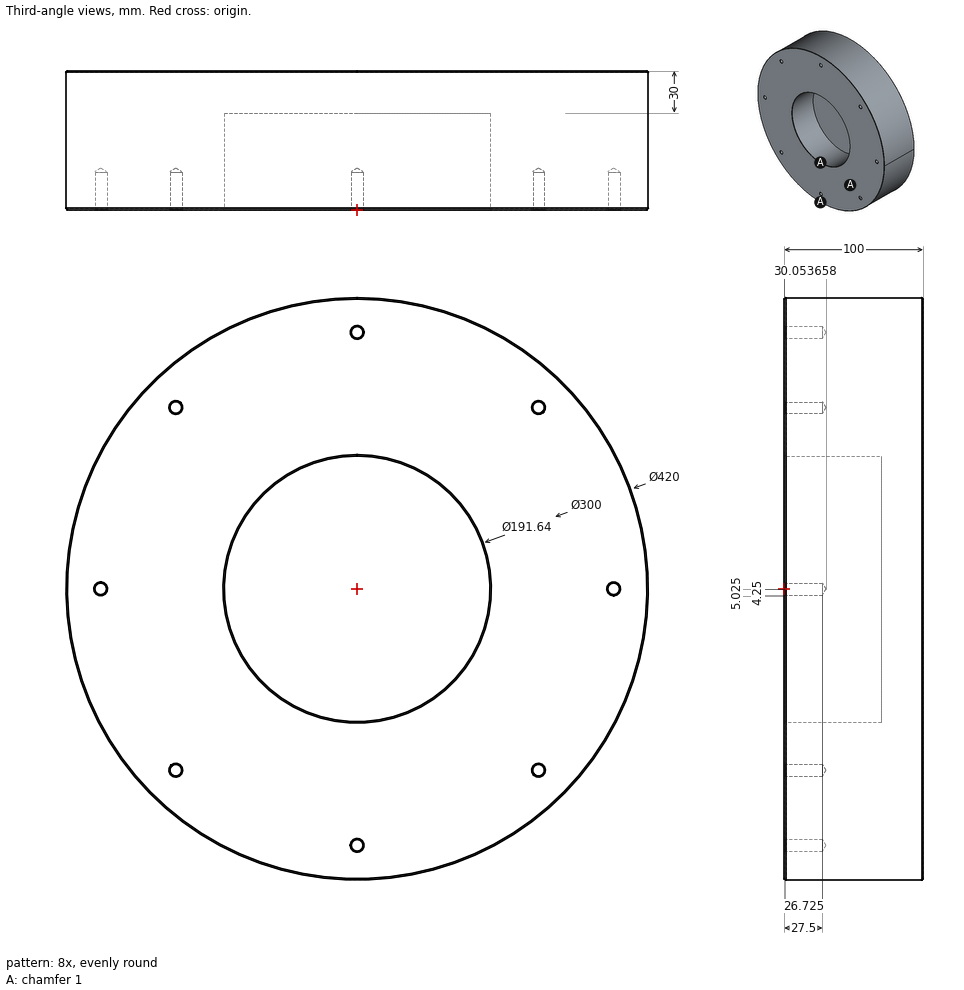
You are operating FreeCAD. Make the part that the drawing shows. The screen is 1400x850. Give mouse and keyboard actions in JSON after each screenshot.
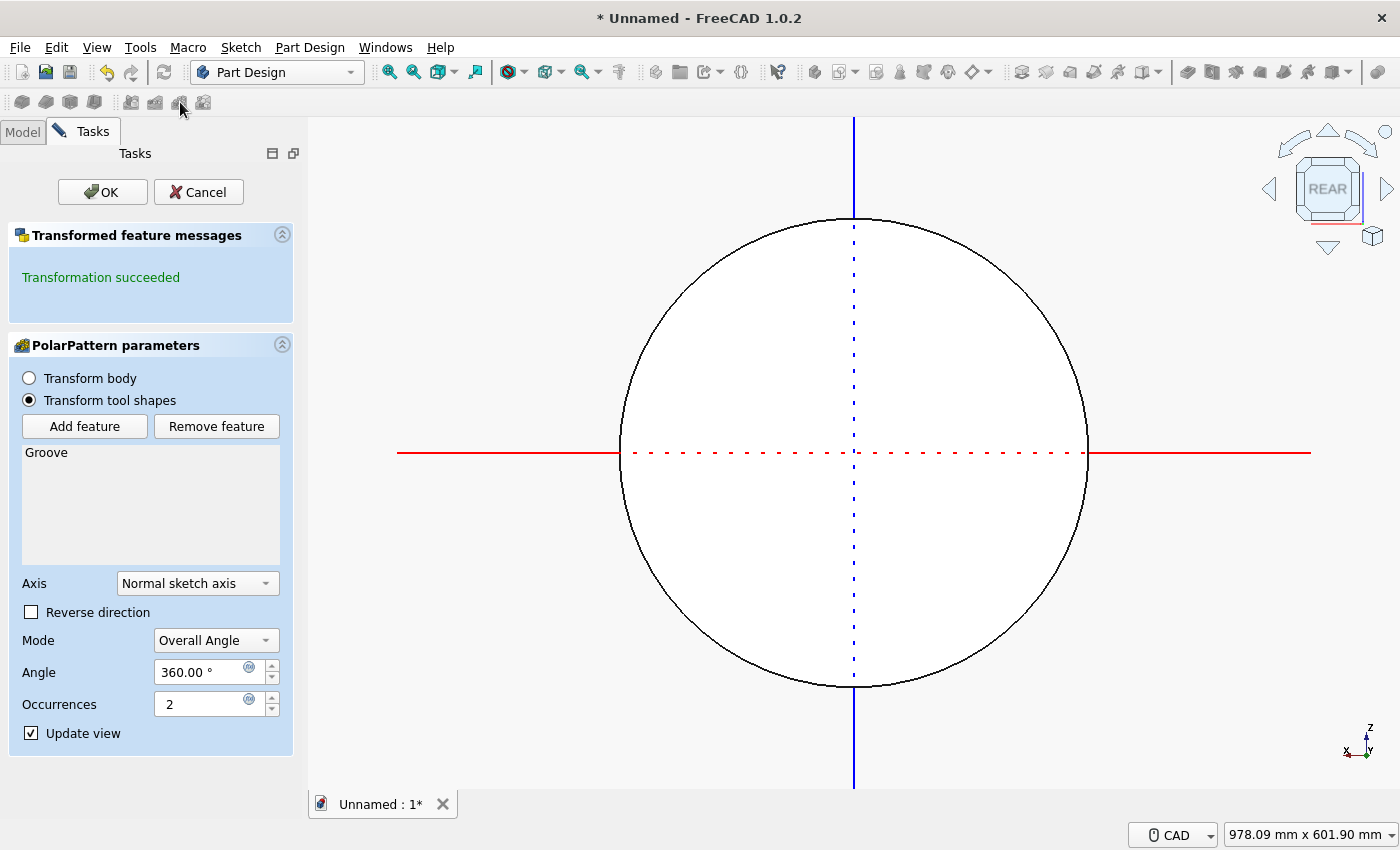
{"action": "left_click", "coordinate": [198, 584]}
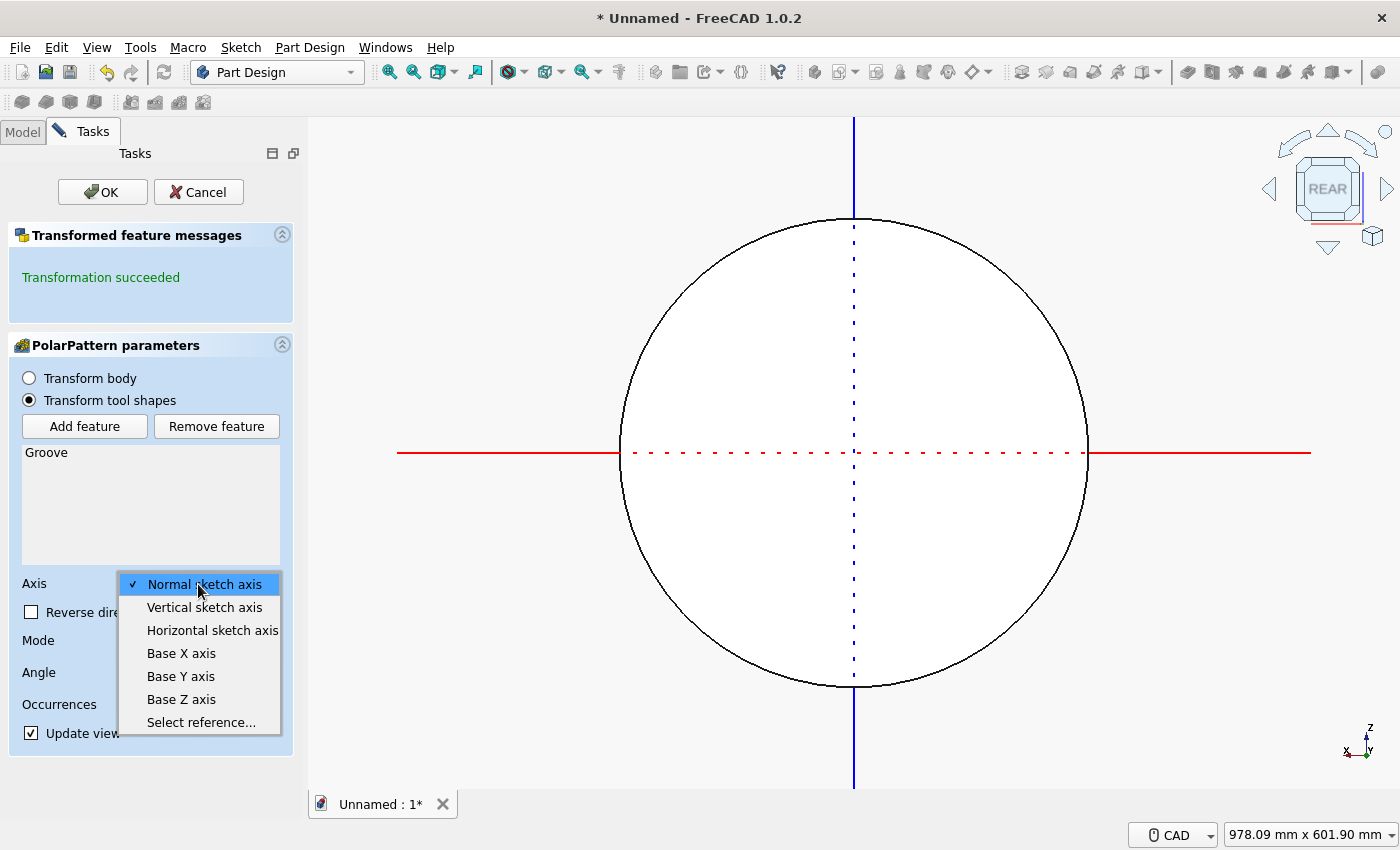
{"action": "left_click", "coordinate": [198, 676]}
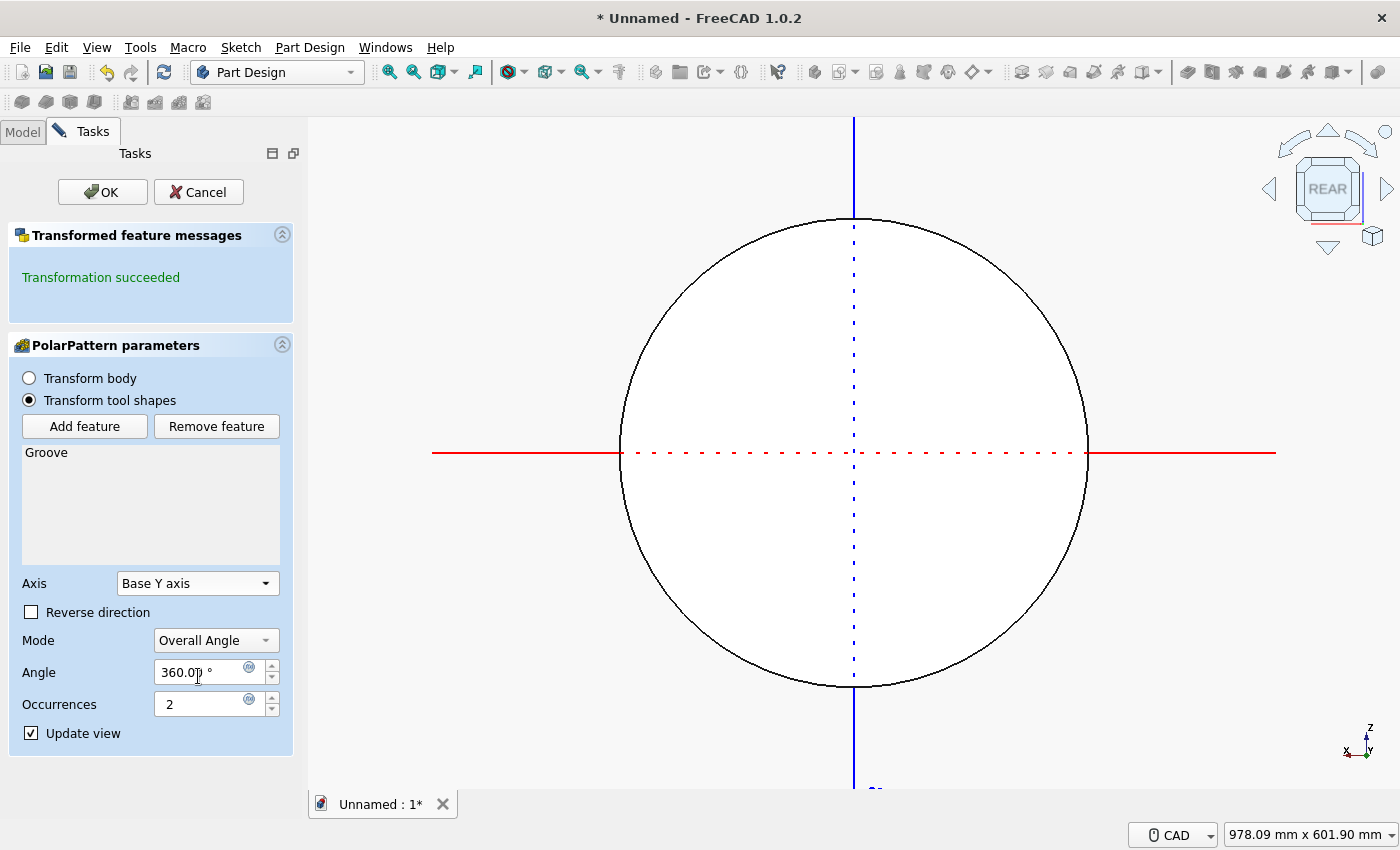
{"action": "triple_click", "coordinate": [209, 704]}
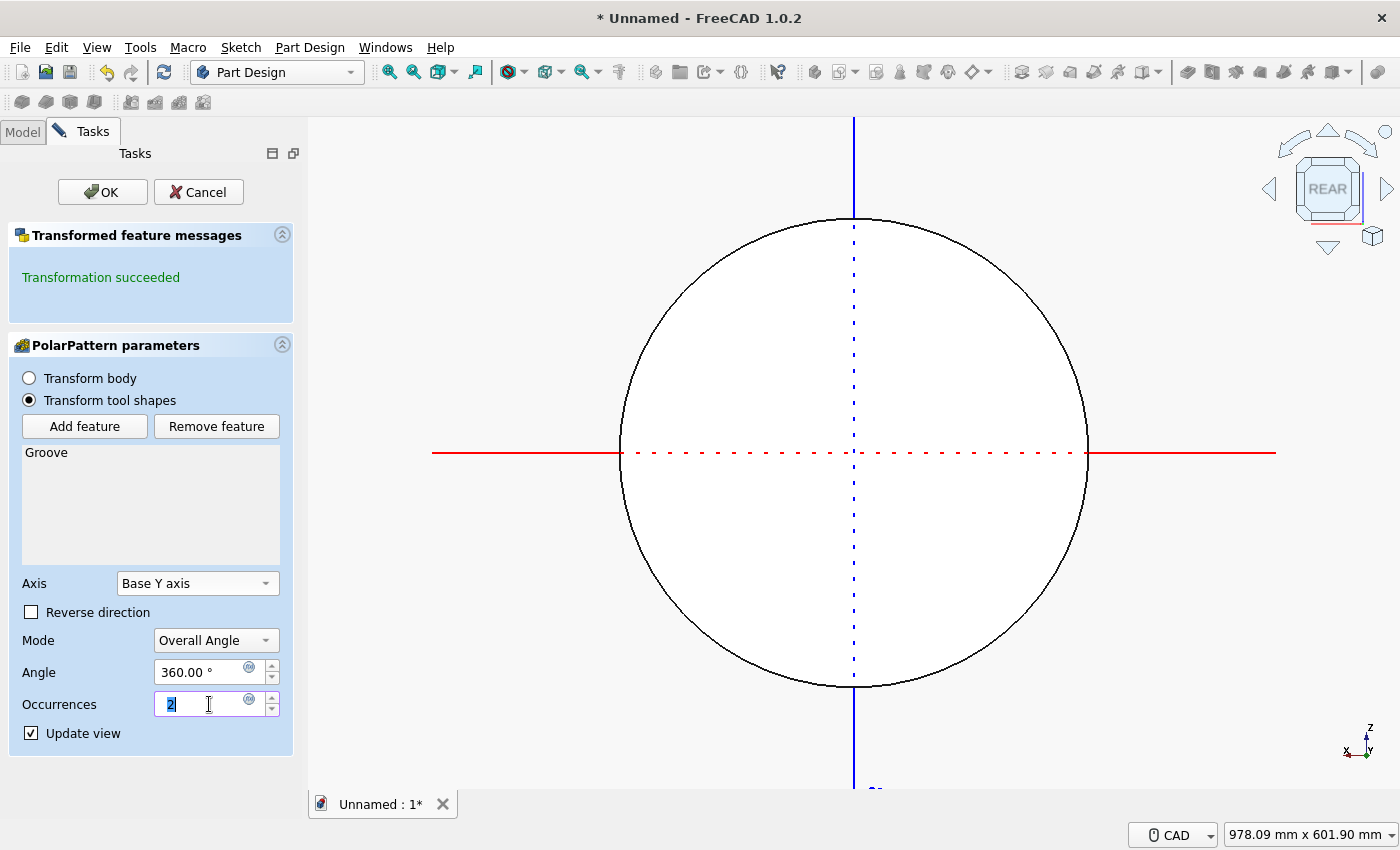
{"action": "type", "text": "8"}
{"action": "key", "text": "Tab"}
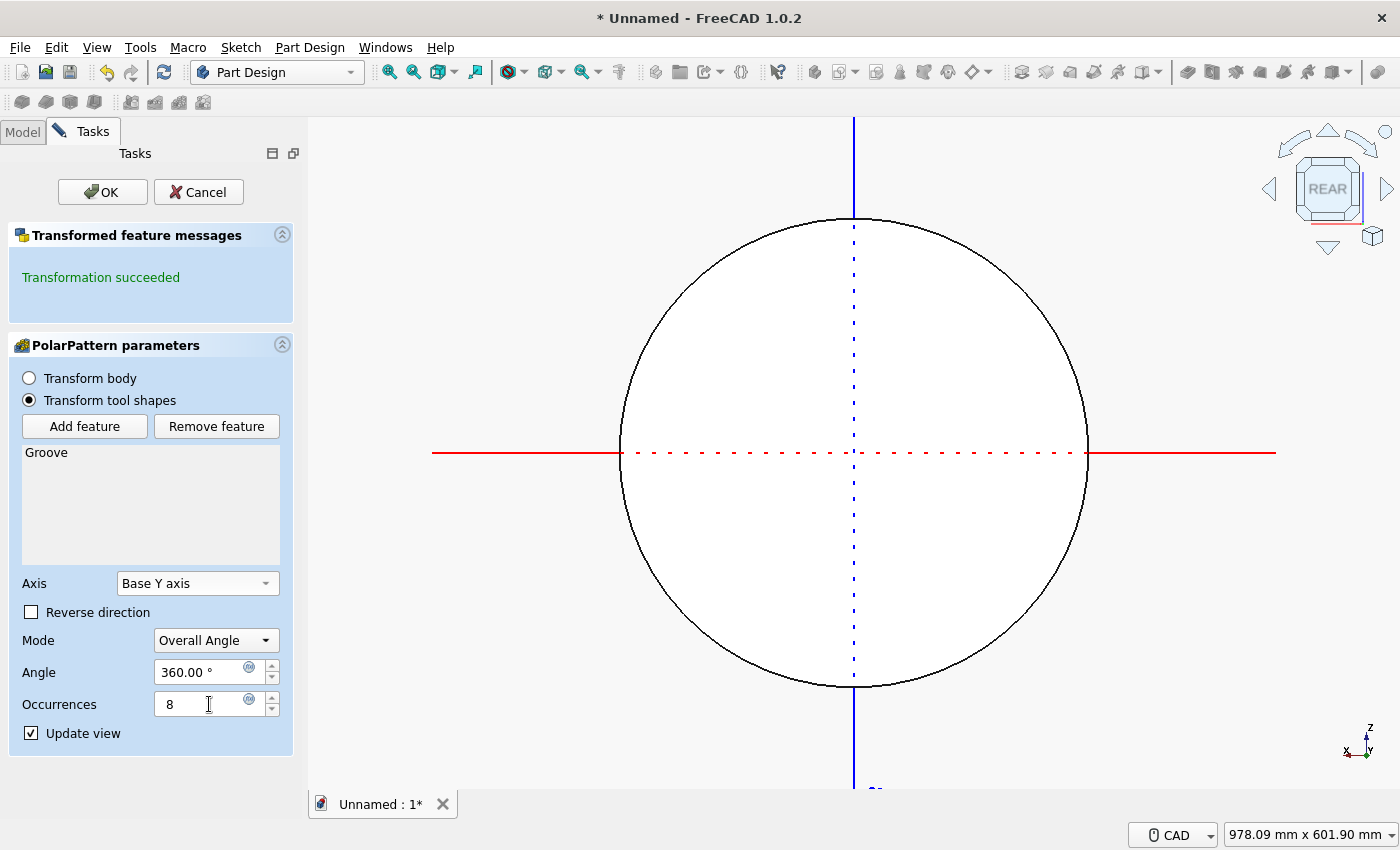
{"action": "left_click", "coordinate": [103, 192]}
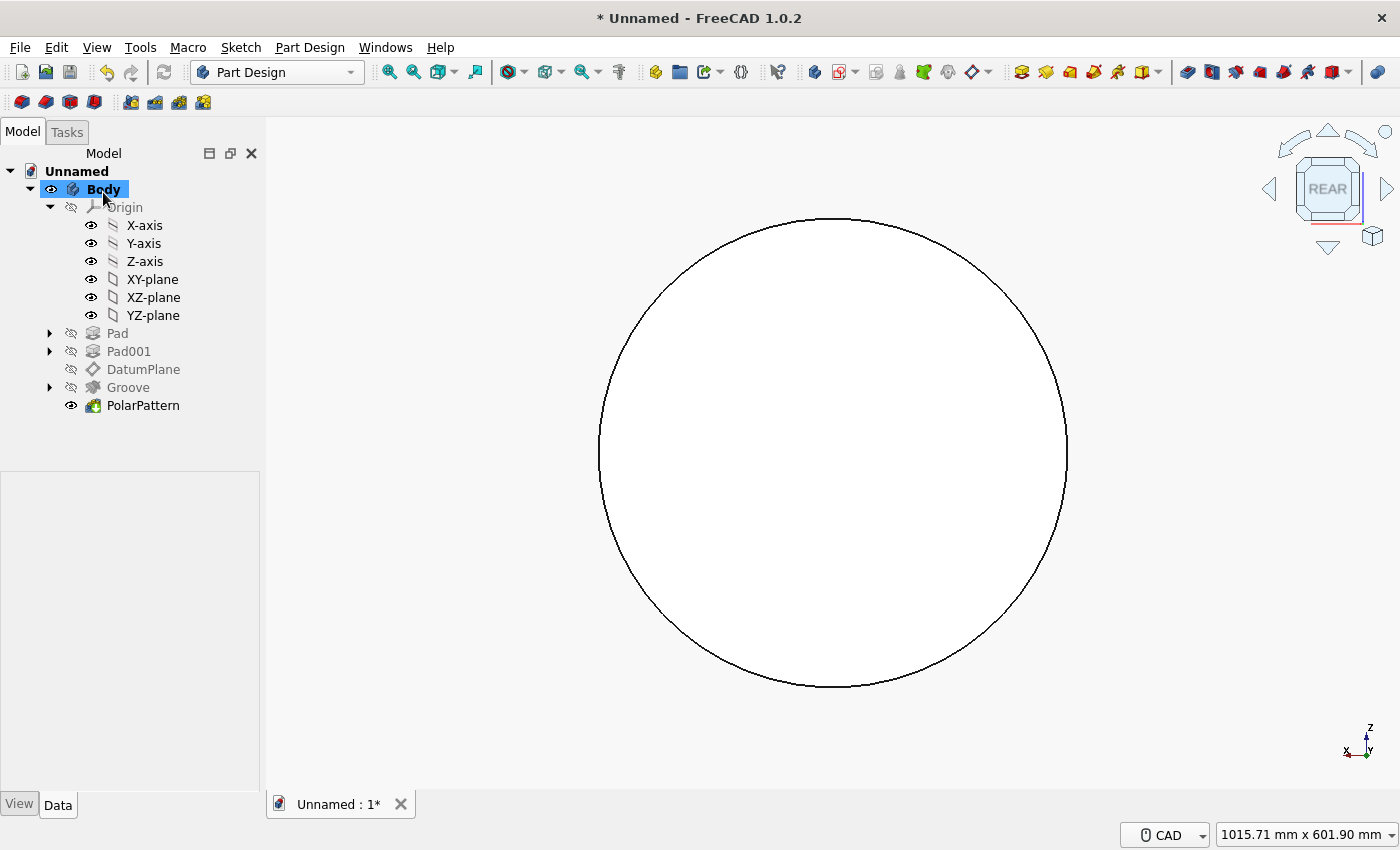
{"action": "left_click", "coordinate": [1067, 452]}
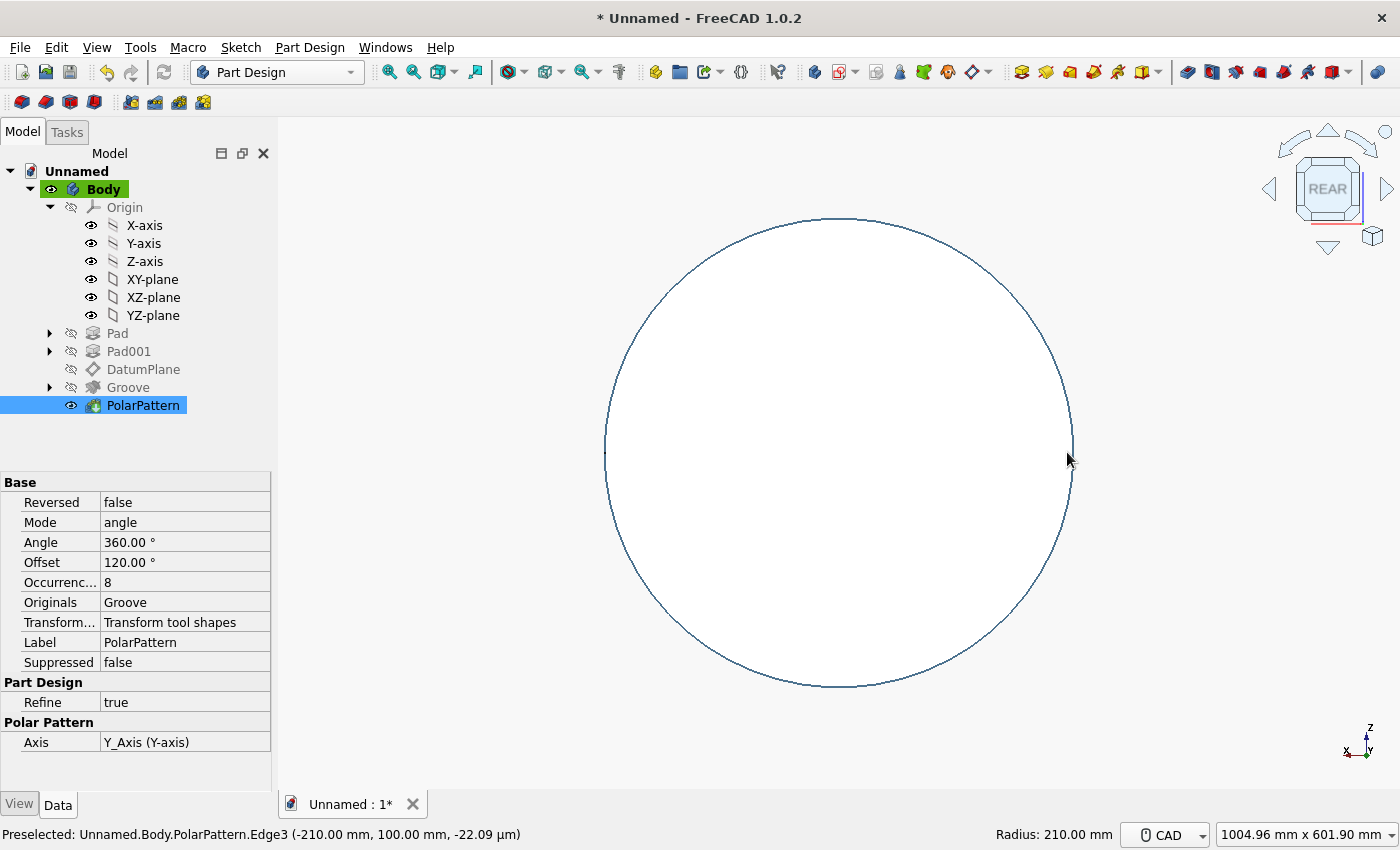
{"action": "key", "text": "0"}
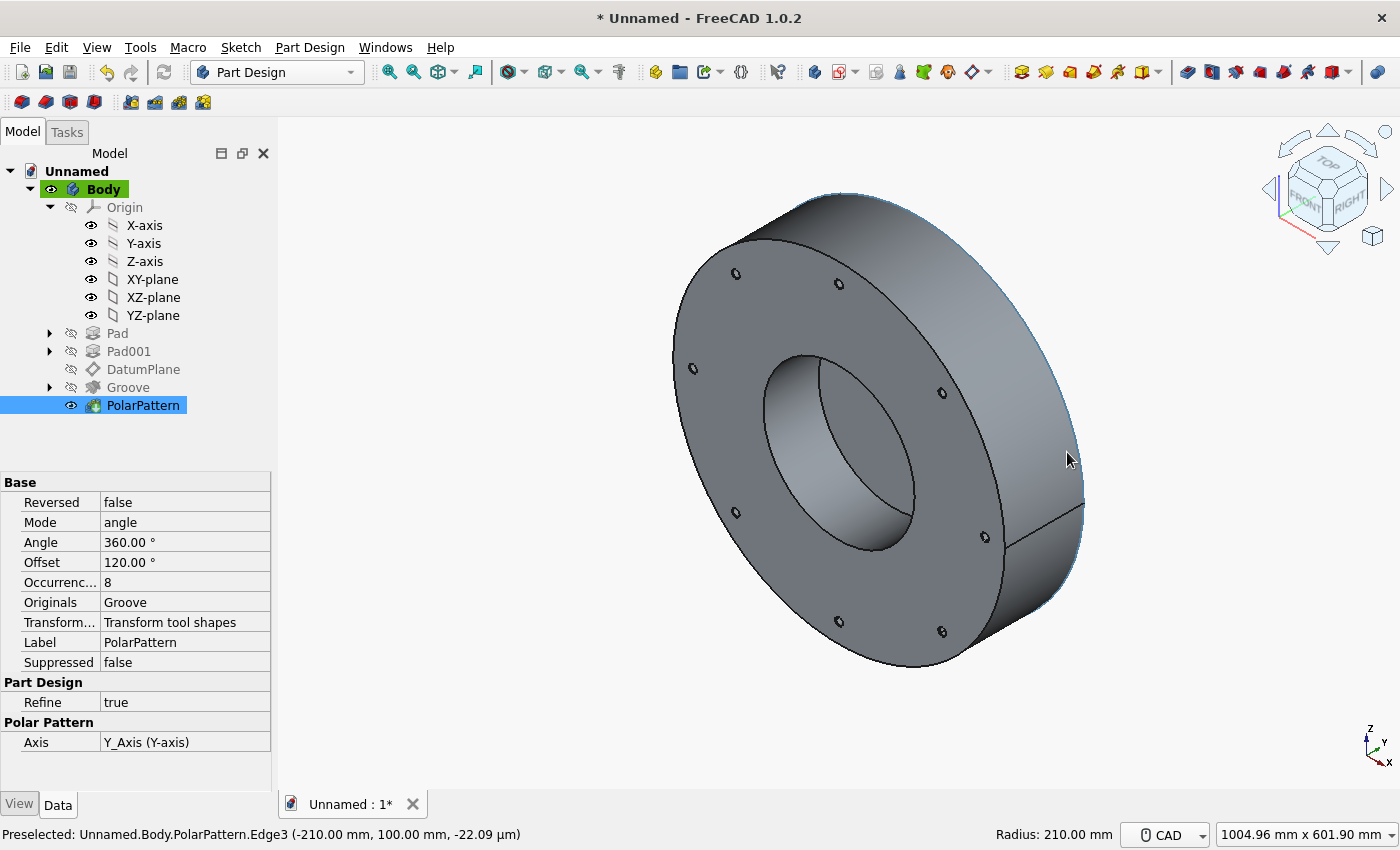
{"action": "left_click", "coordinate": [705, 262], "text": "ctrl"}